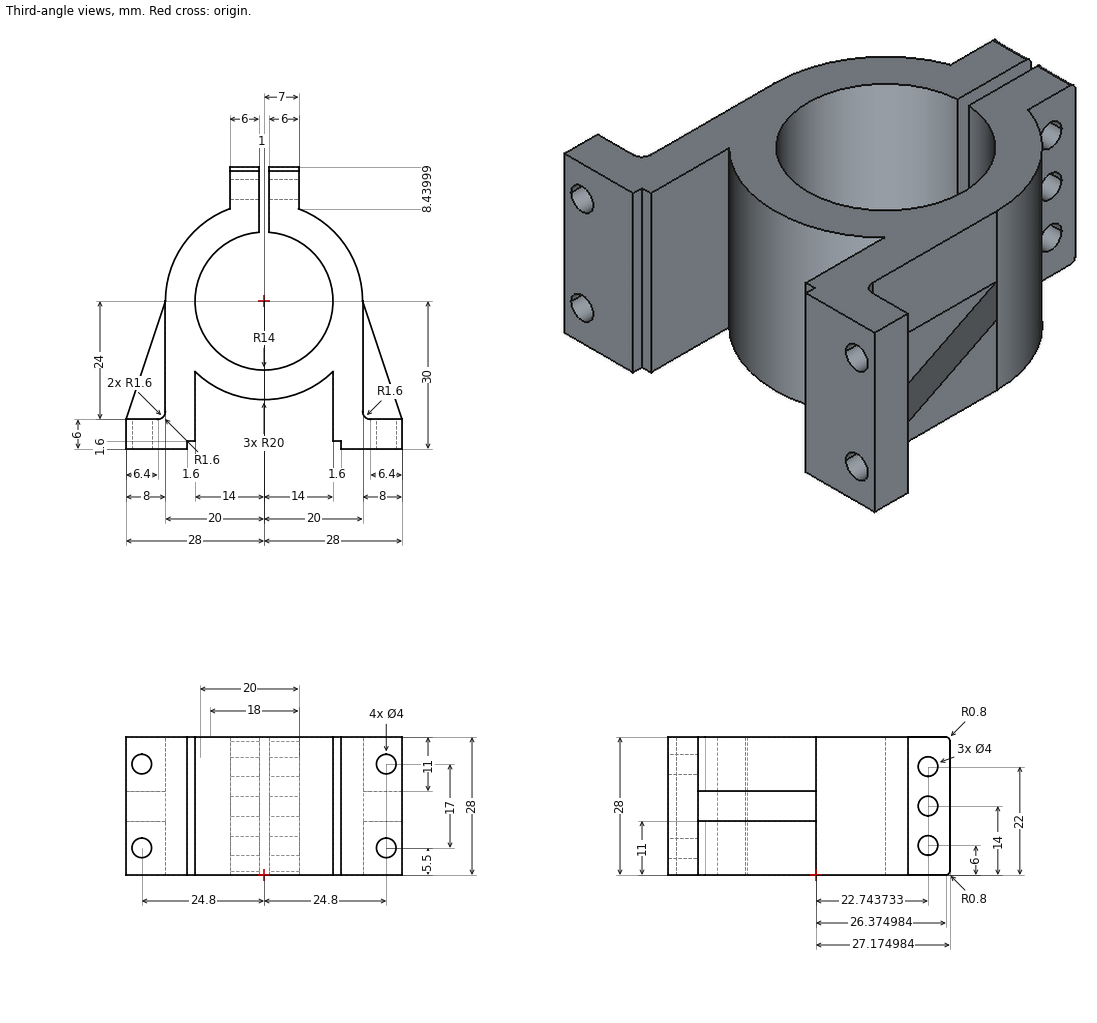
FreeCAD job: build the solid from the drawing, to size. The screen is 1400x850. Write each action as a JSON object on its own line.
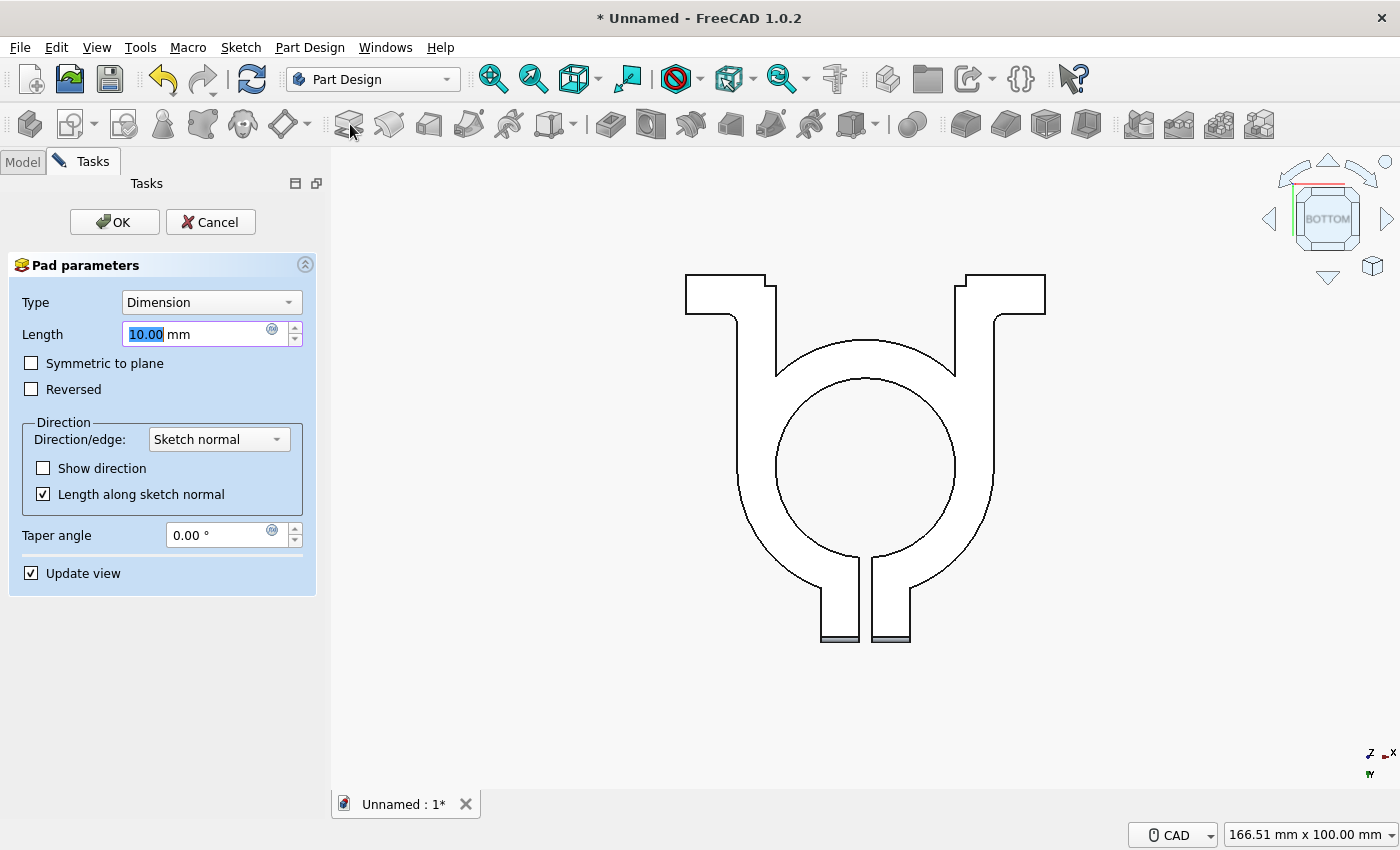
{"action": "type", "text": "28"}
{"action": "key", "text": "Tab"}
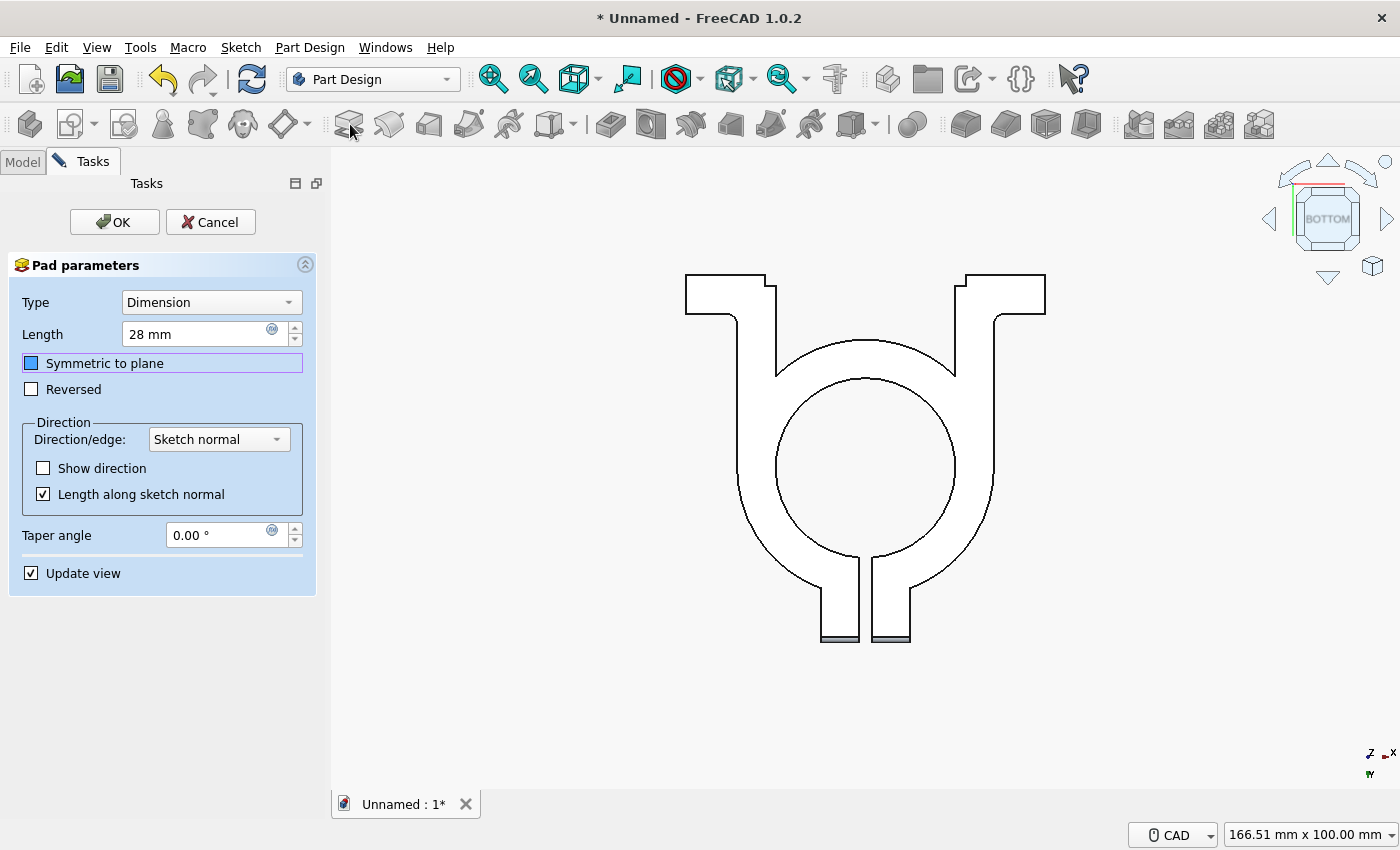
{"action": "left_click", "coordinate": [30, 389]}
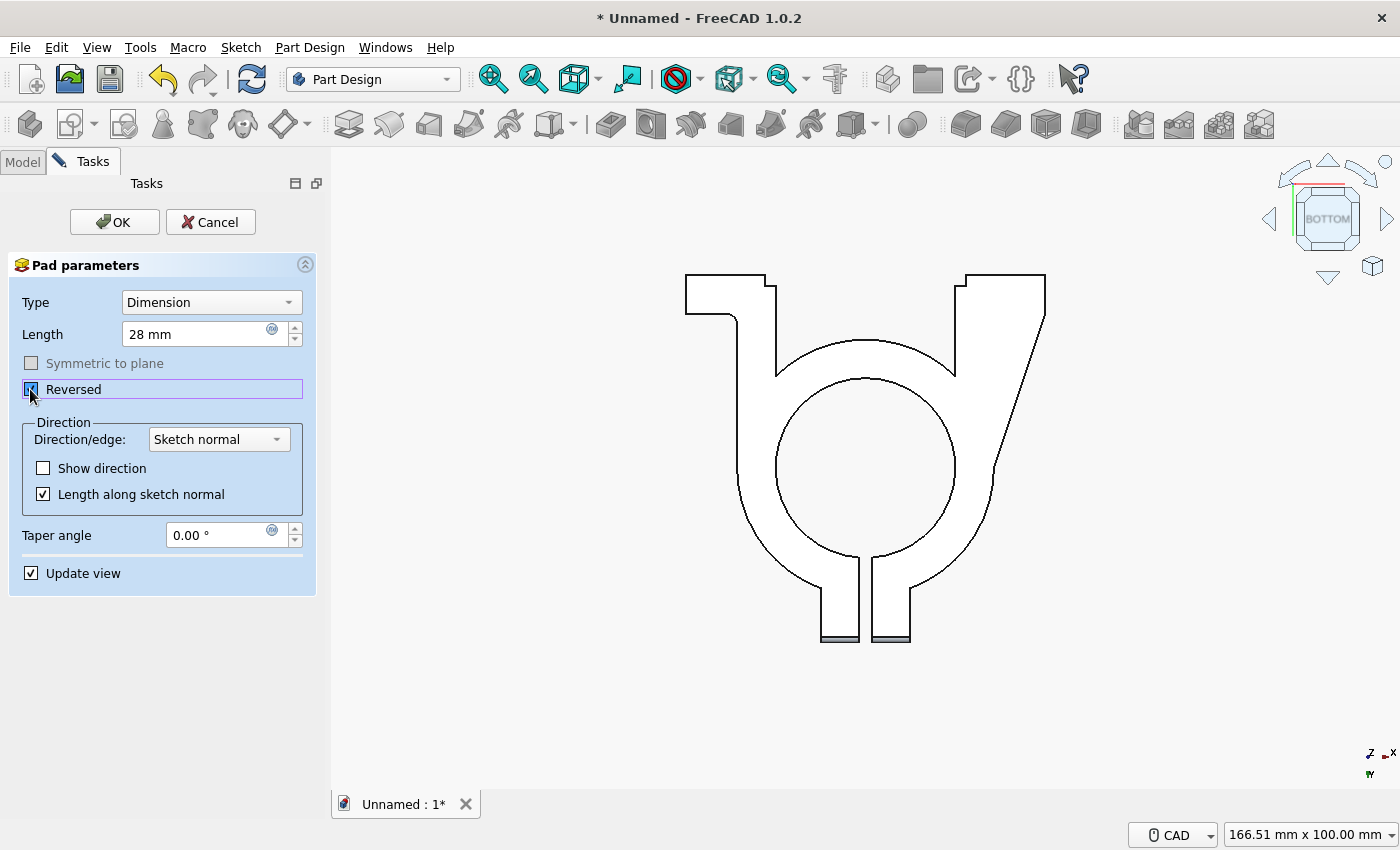
{"action": "left_click", "coordinate": [115, 222]}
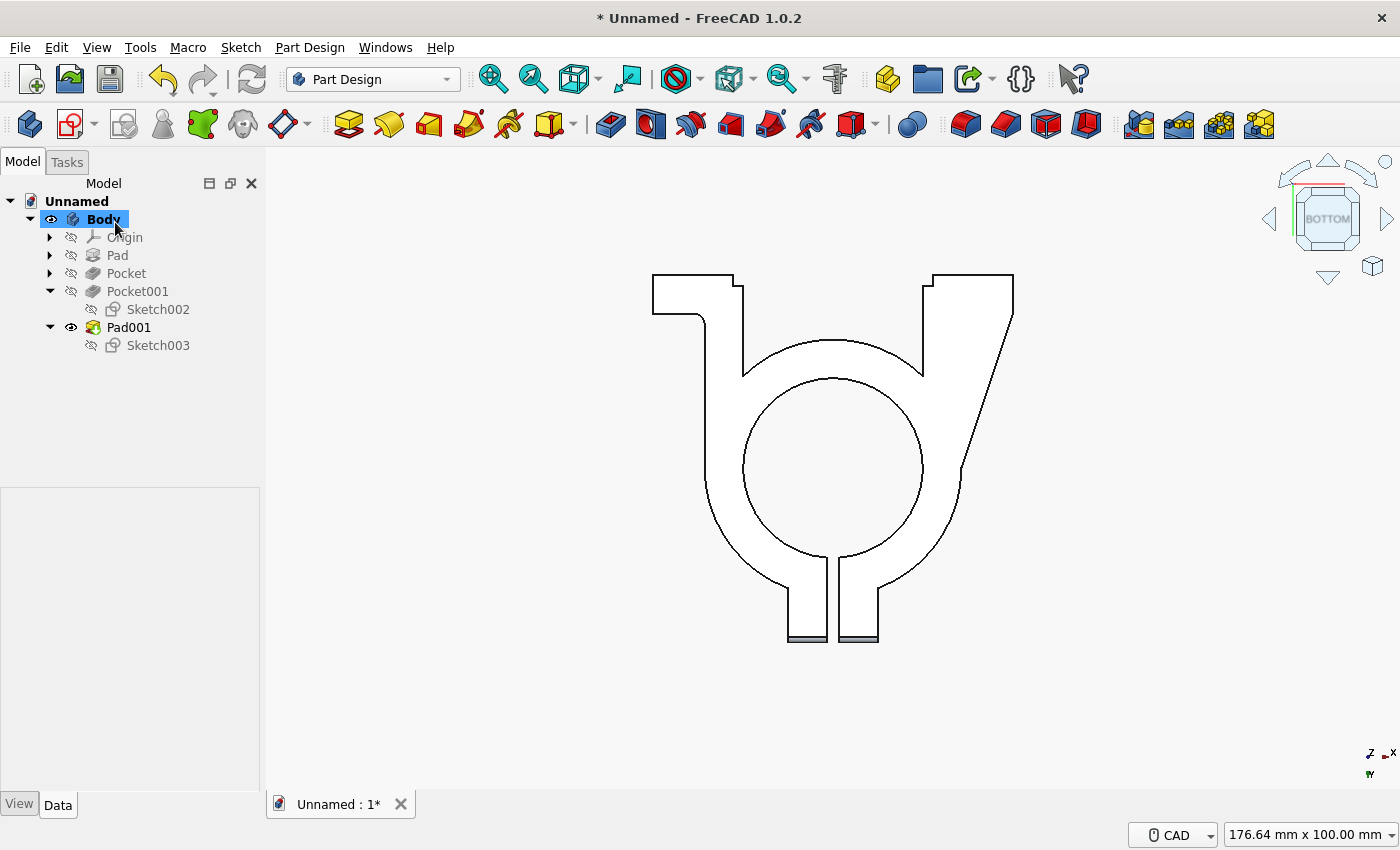
{"action": "key", "text": "0"}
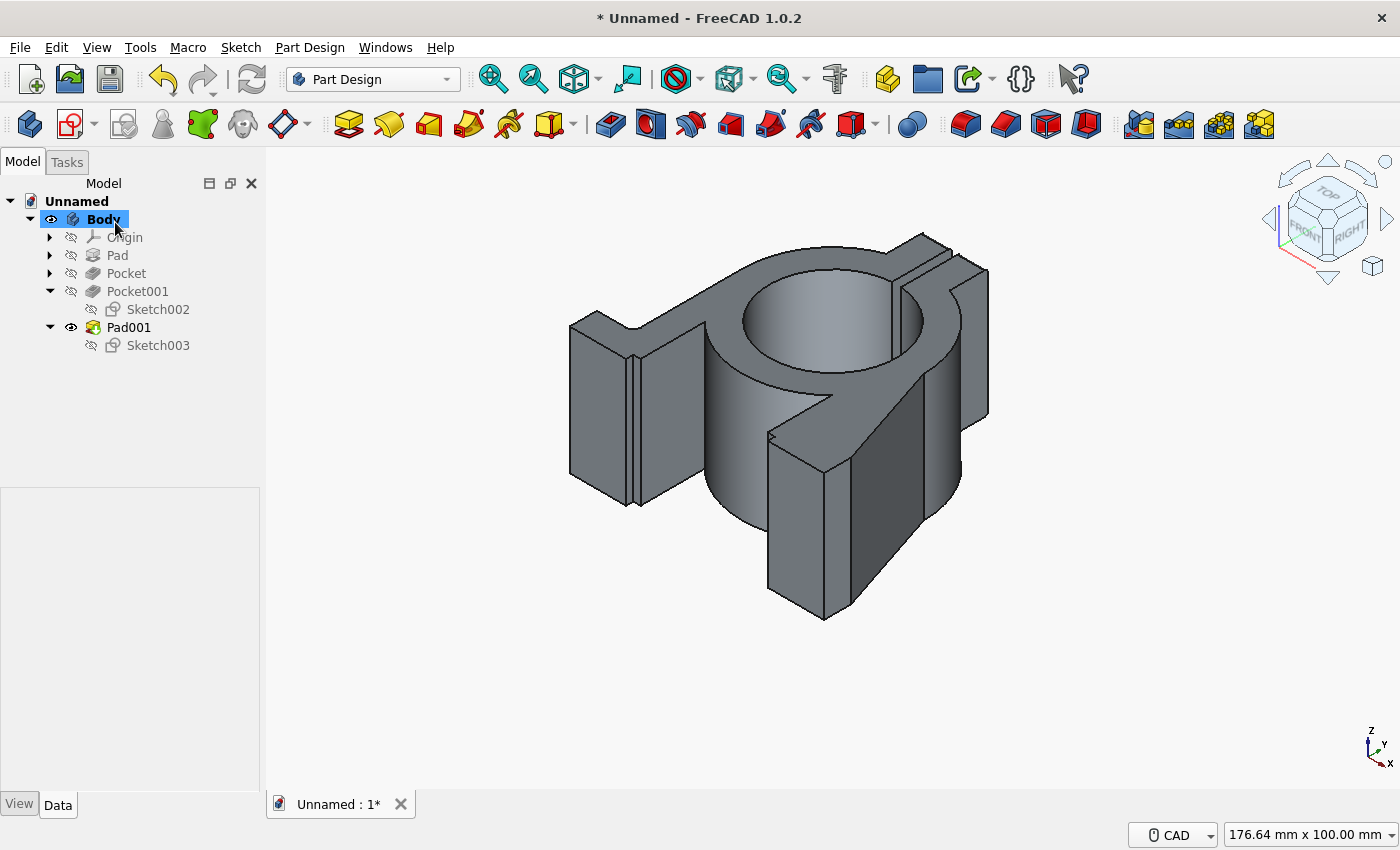
{"action": "left_click", "coordinate": [861, 388]}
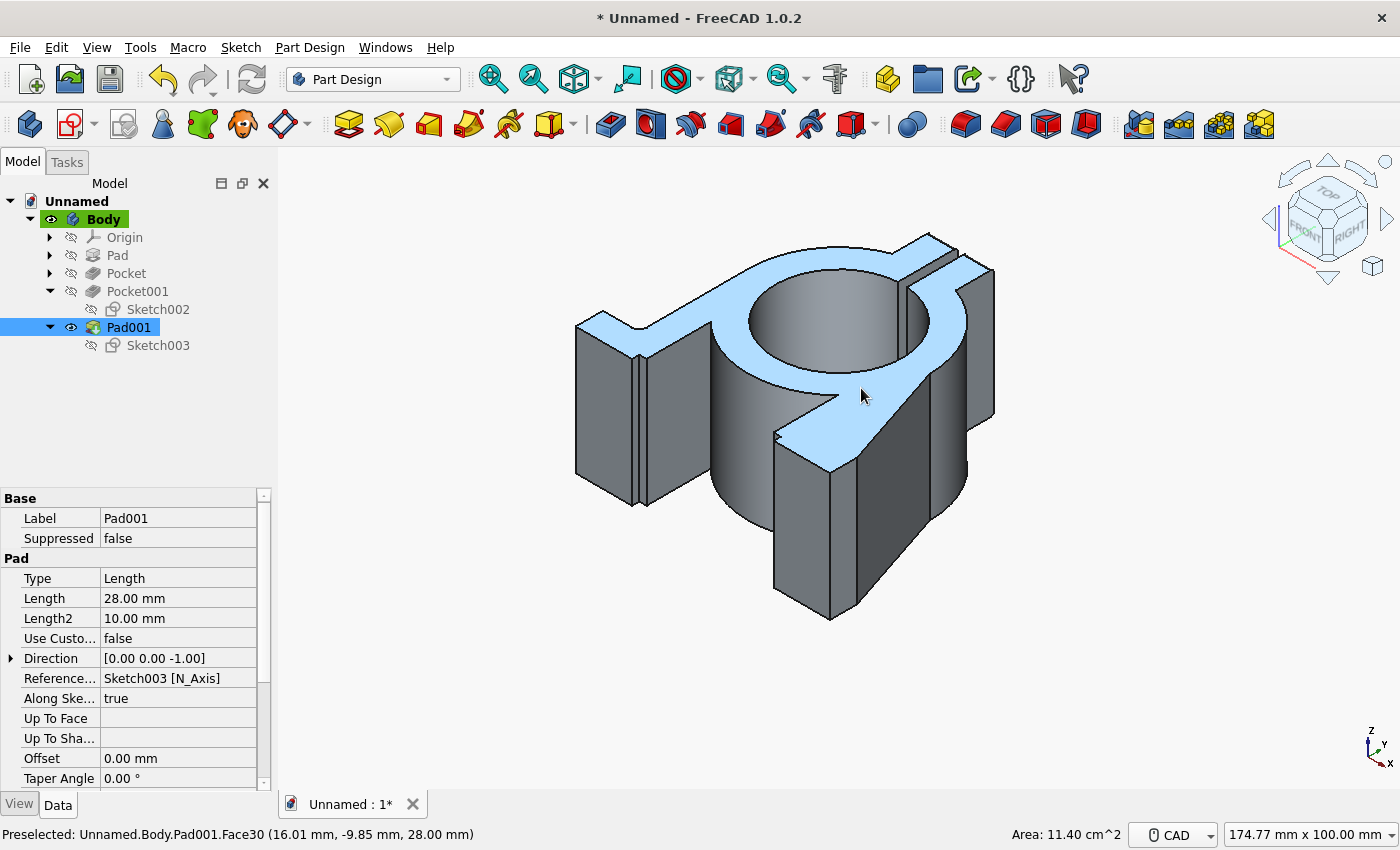
{"action": "left_click", "coordinate": [70, 124]}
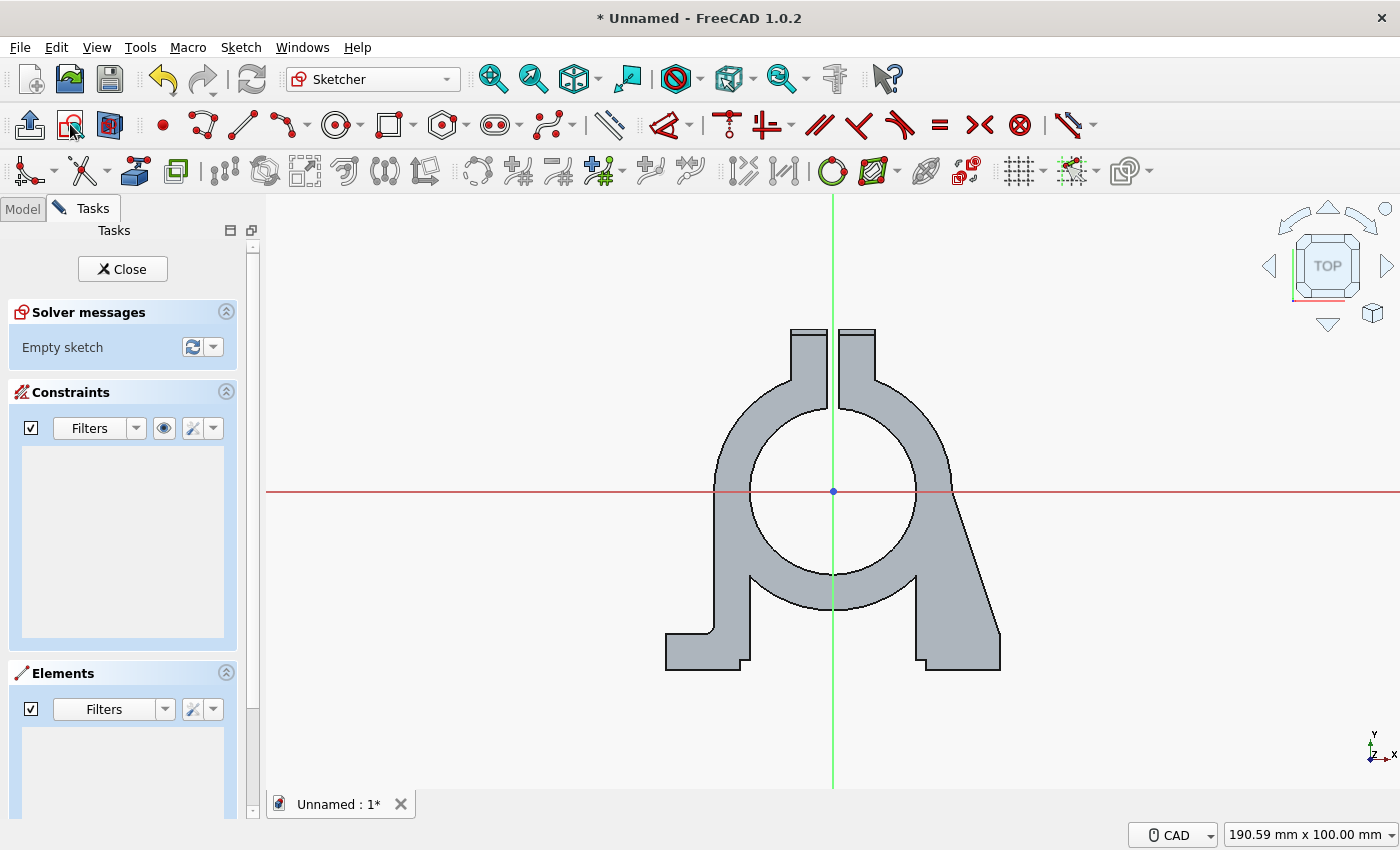
{"action": "scroll", "coordinate": [1005, 604], "scroll_direction": "up", "scroll_amount": 5}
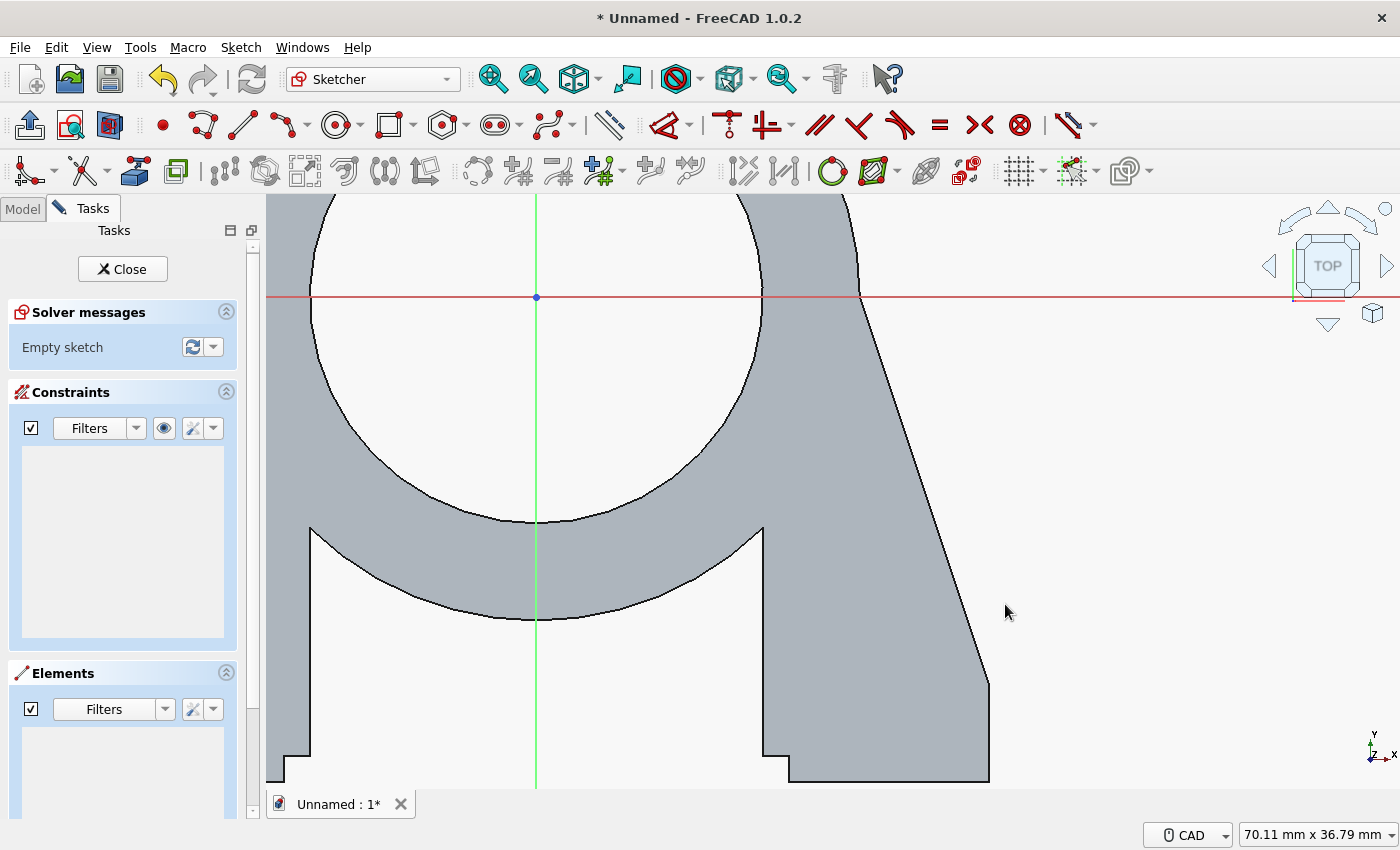
{"action": "left_click", "coordinate": [204, 126]}